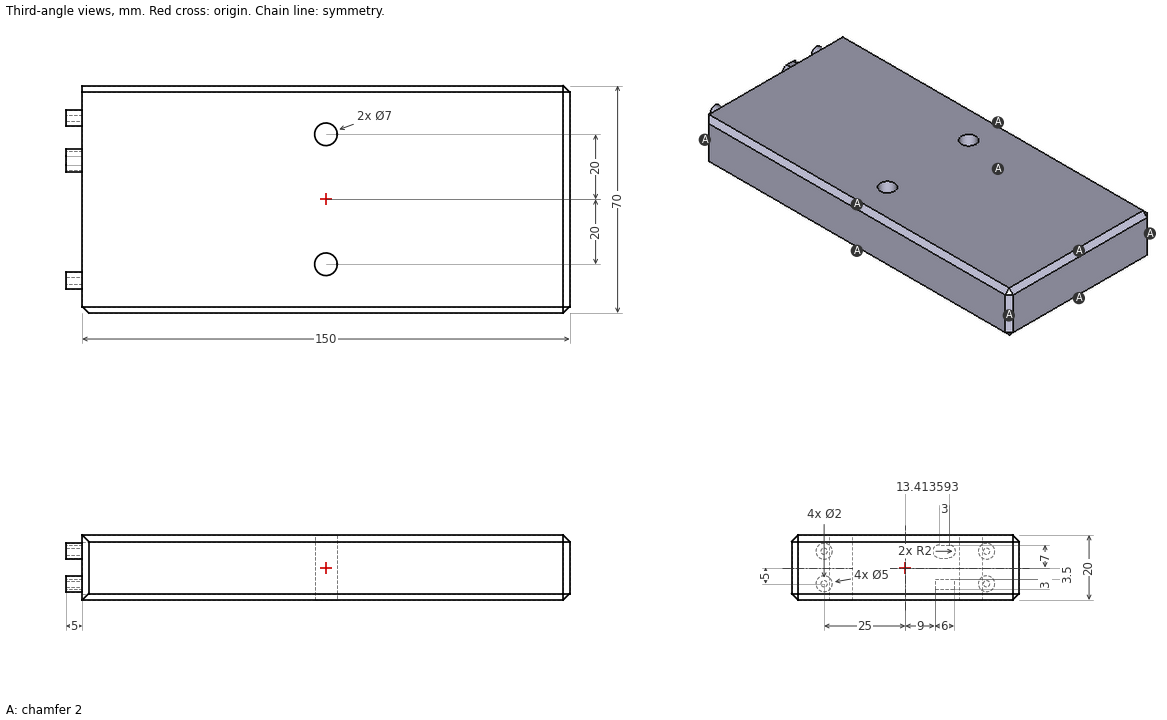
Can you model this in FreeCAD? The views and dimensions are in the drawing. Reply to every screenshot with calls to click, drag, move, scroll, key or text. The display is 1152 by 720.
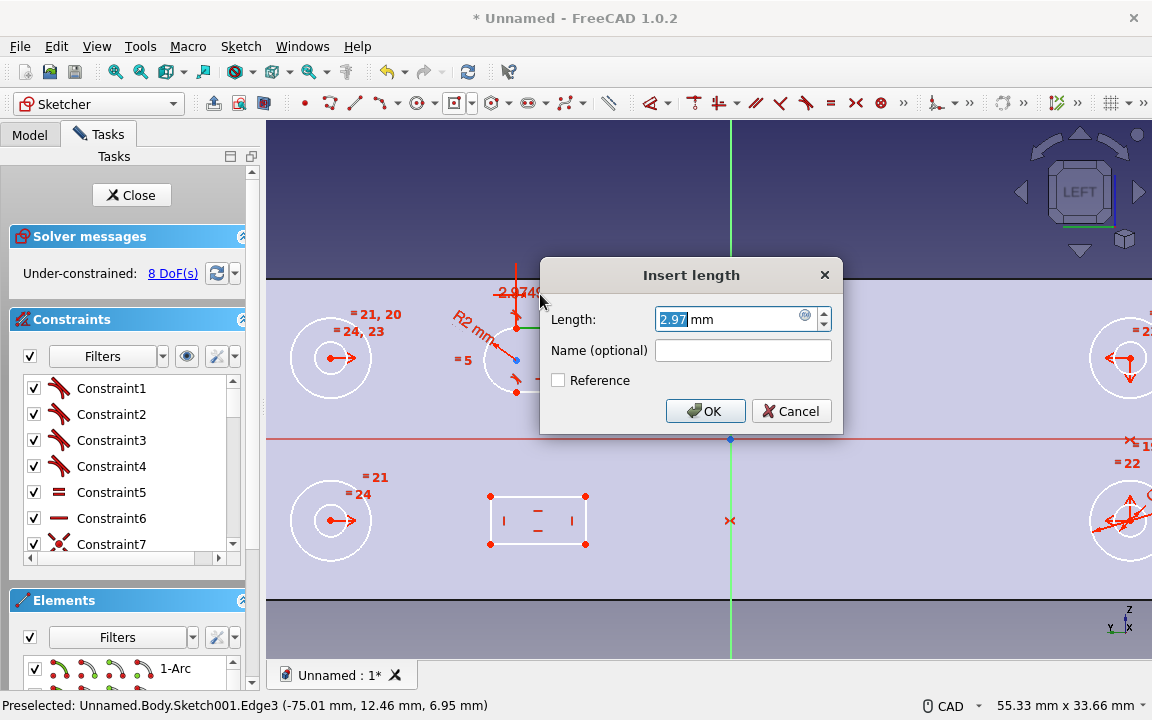
text(3)
key(Return)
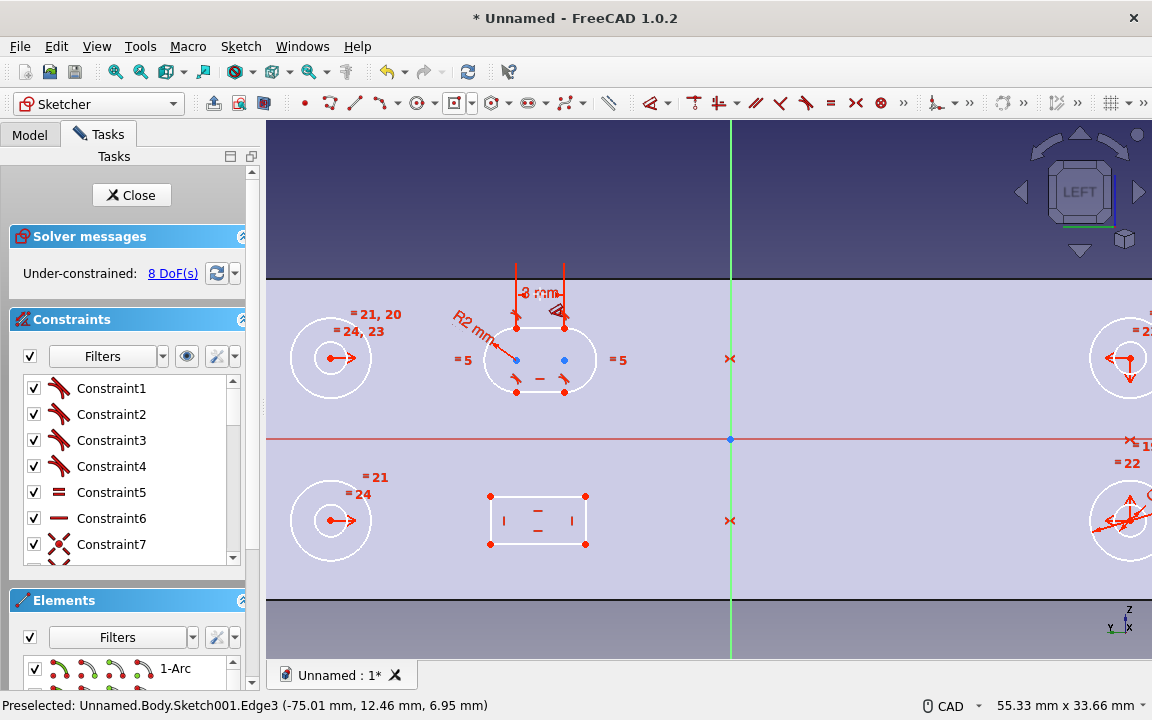
click(491, 511)
click(457, 520)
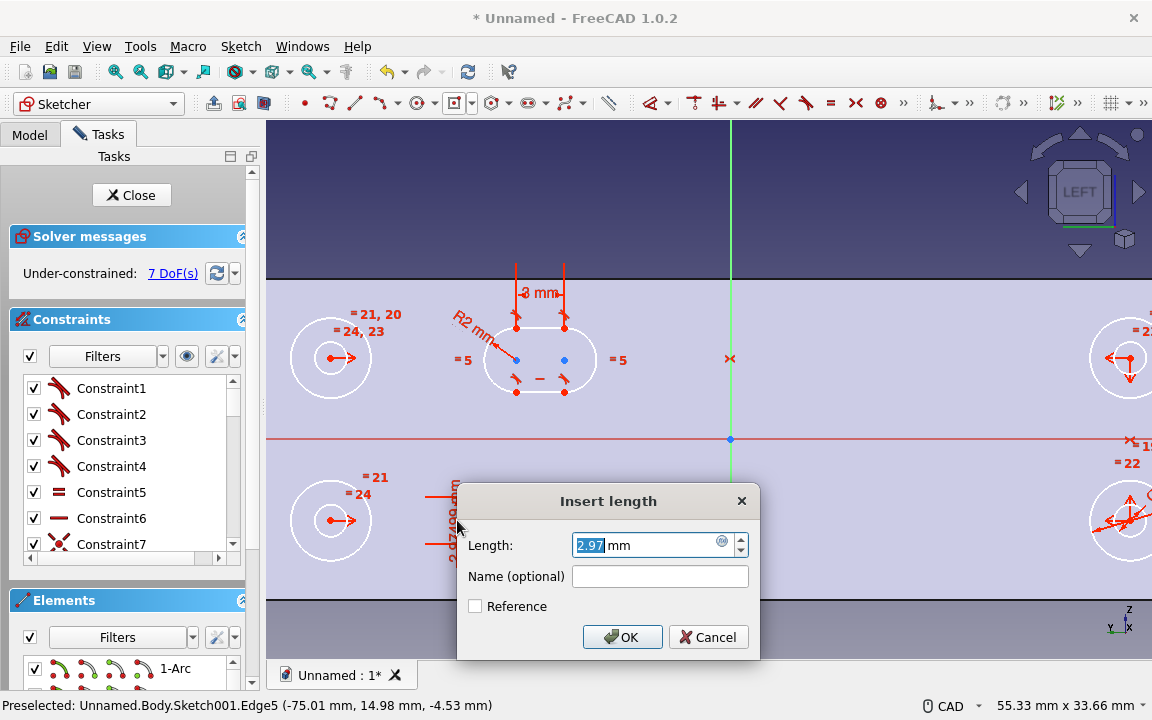
text(3)
key(Return)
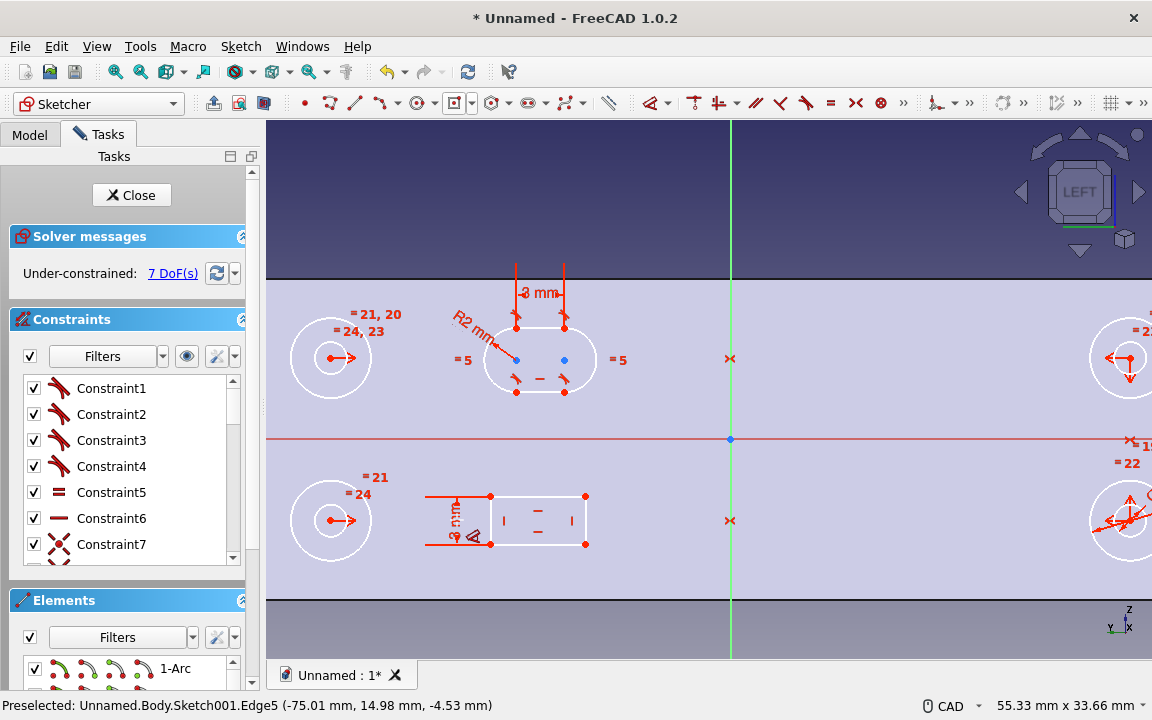
click(519, 545)
click(538, 579)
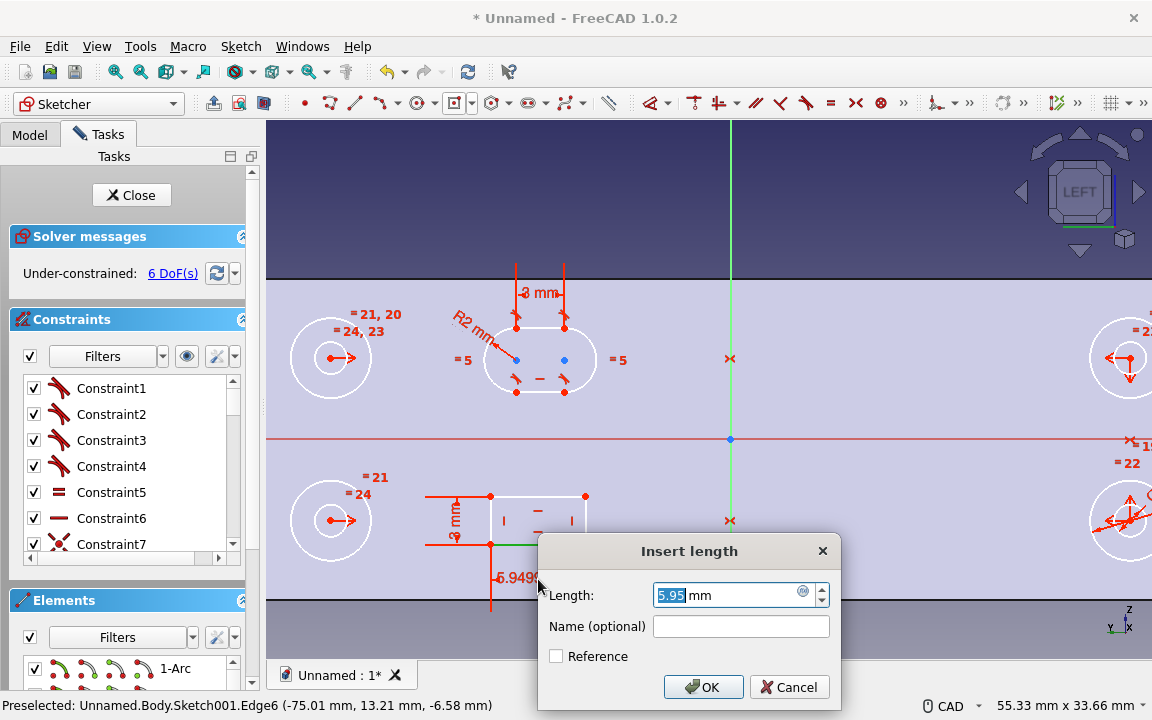
text(6)
key(Return)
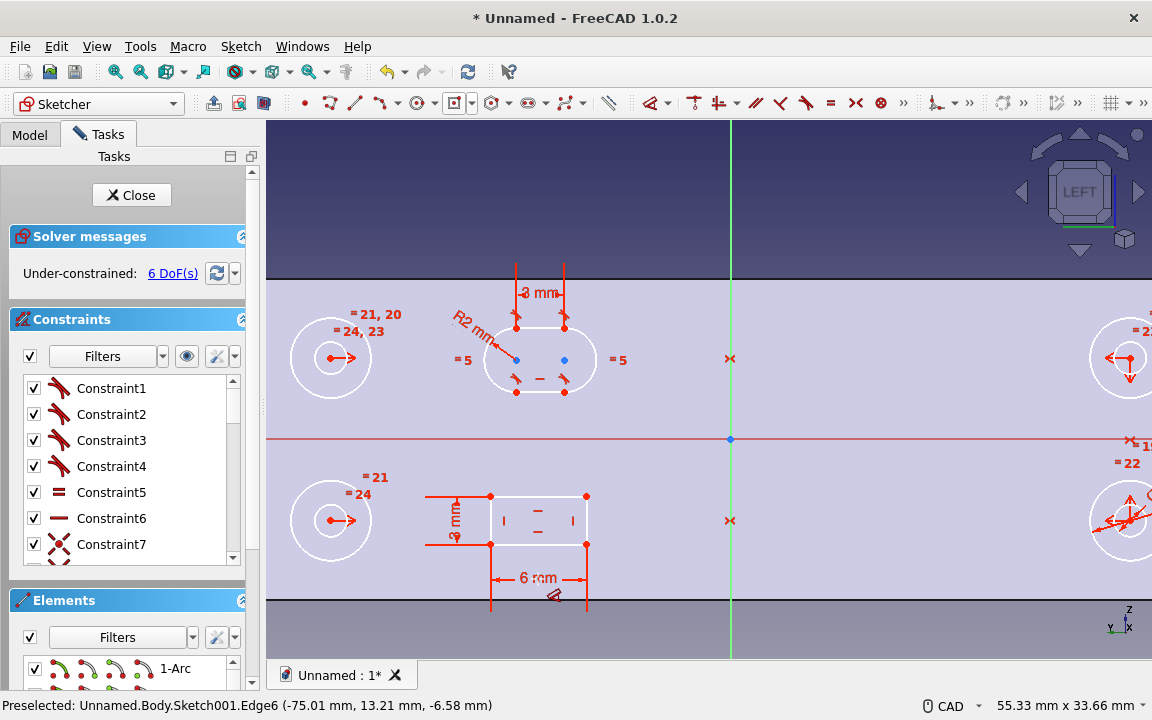
scroll(531, 329, down, 3)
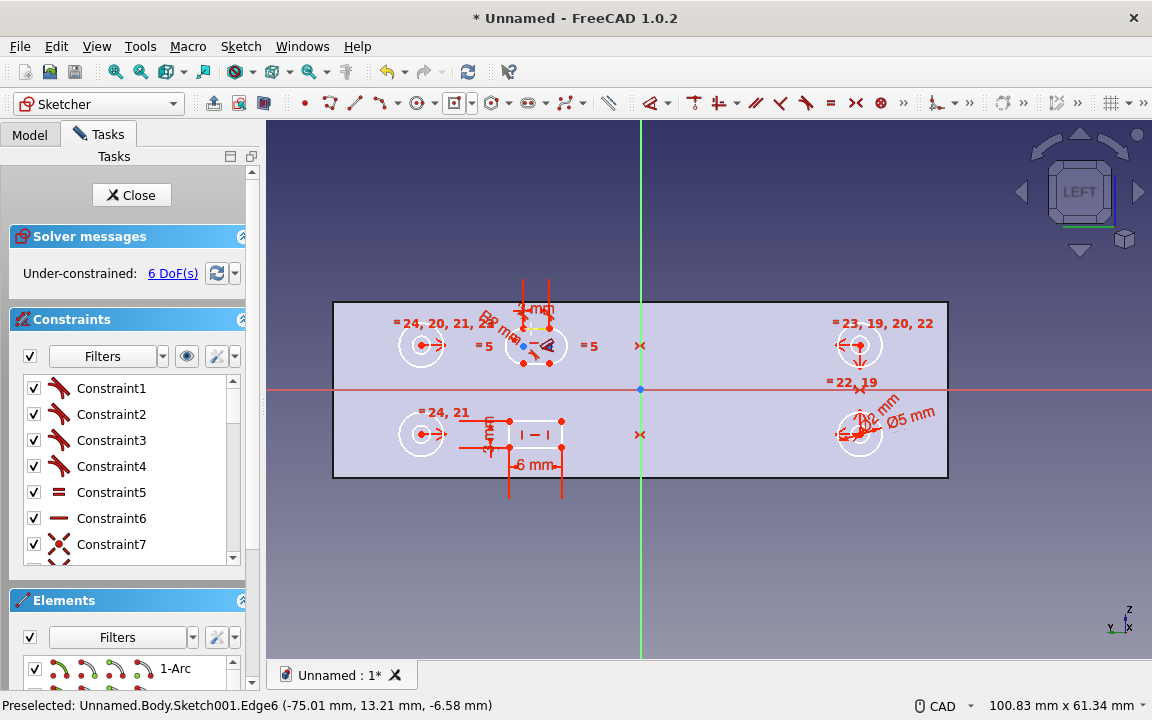
click(860, 434)
click(607, 412)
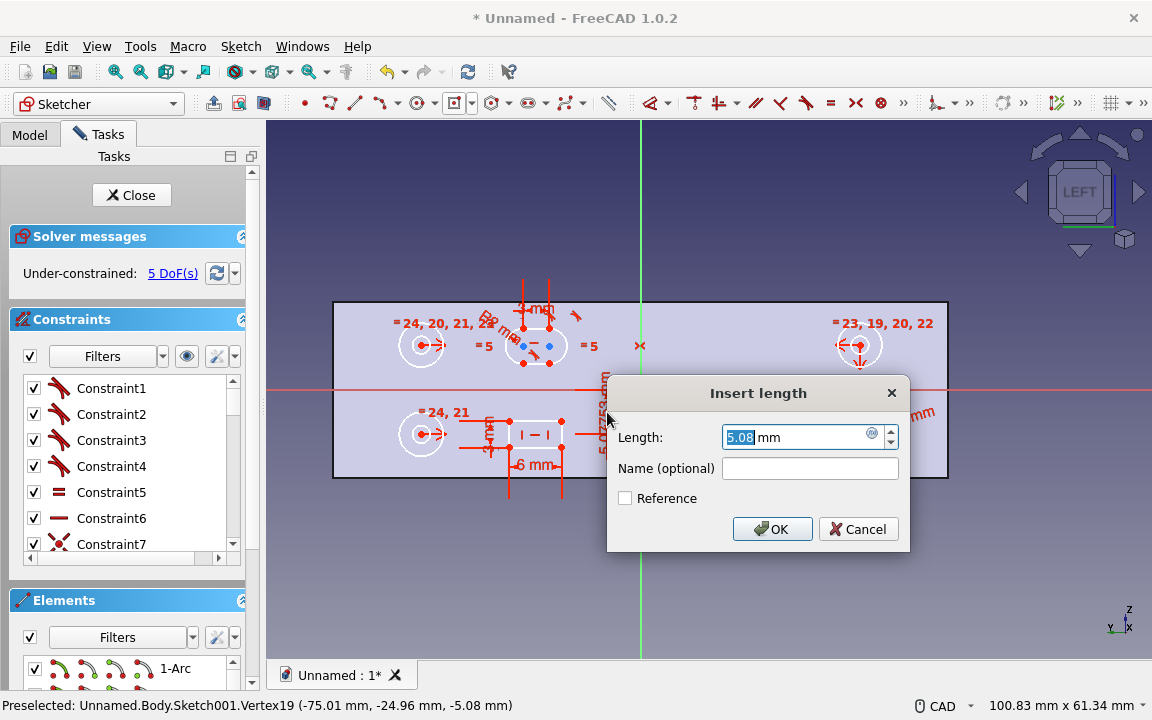
text(5)
key(Return)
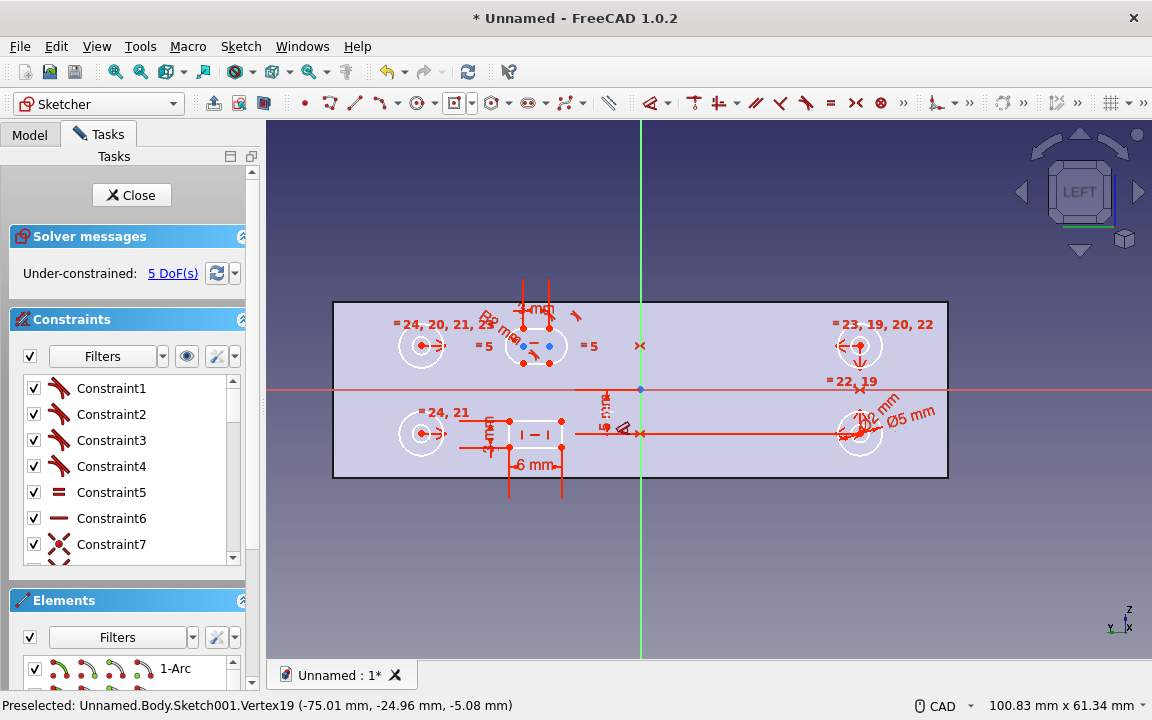
click(523, 329)
click(489, 359)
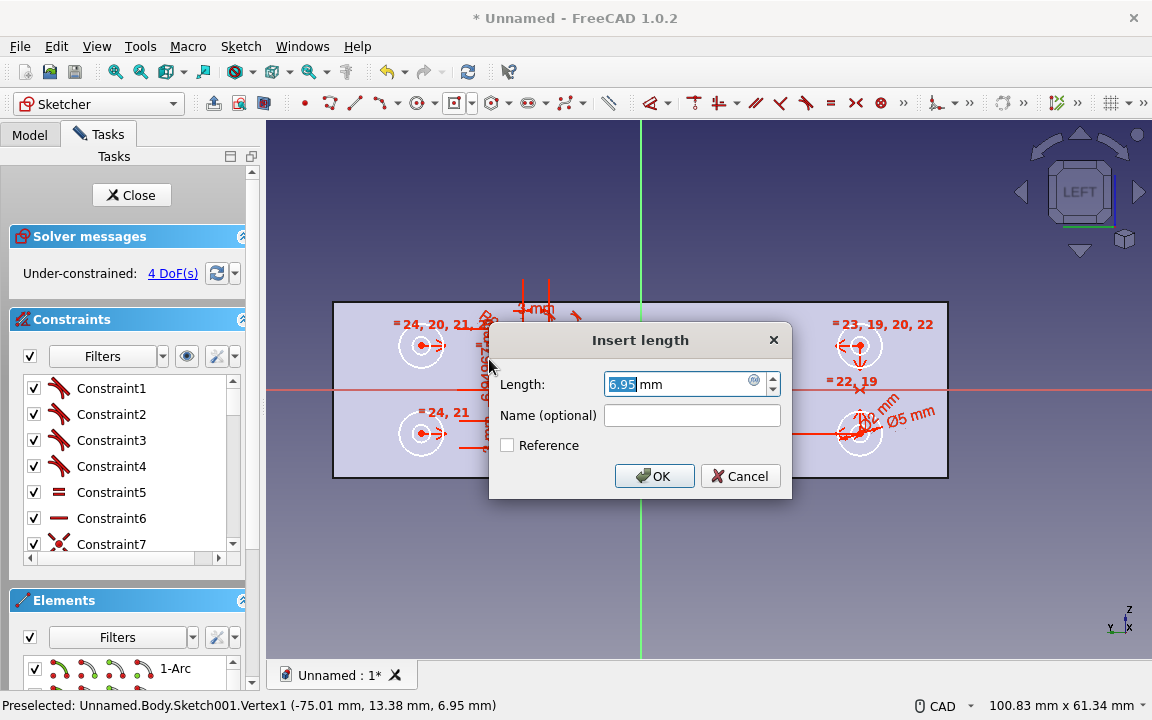
text(7)
key(Return)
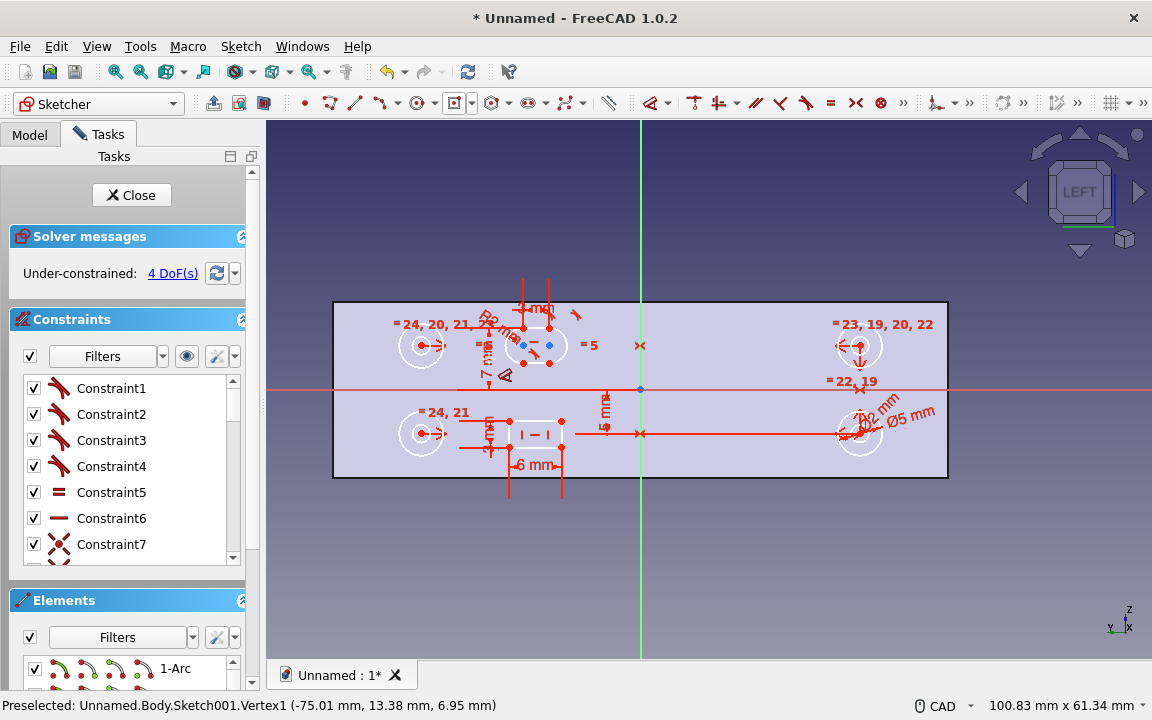
click(562, 448)
click(619, 482)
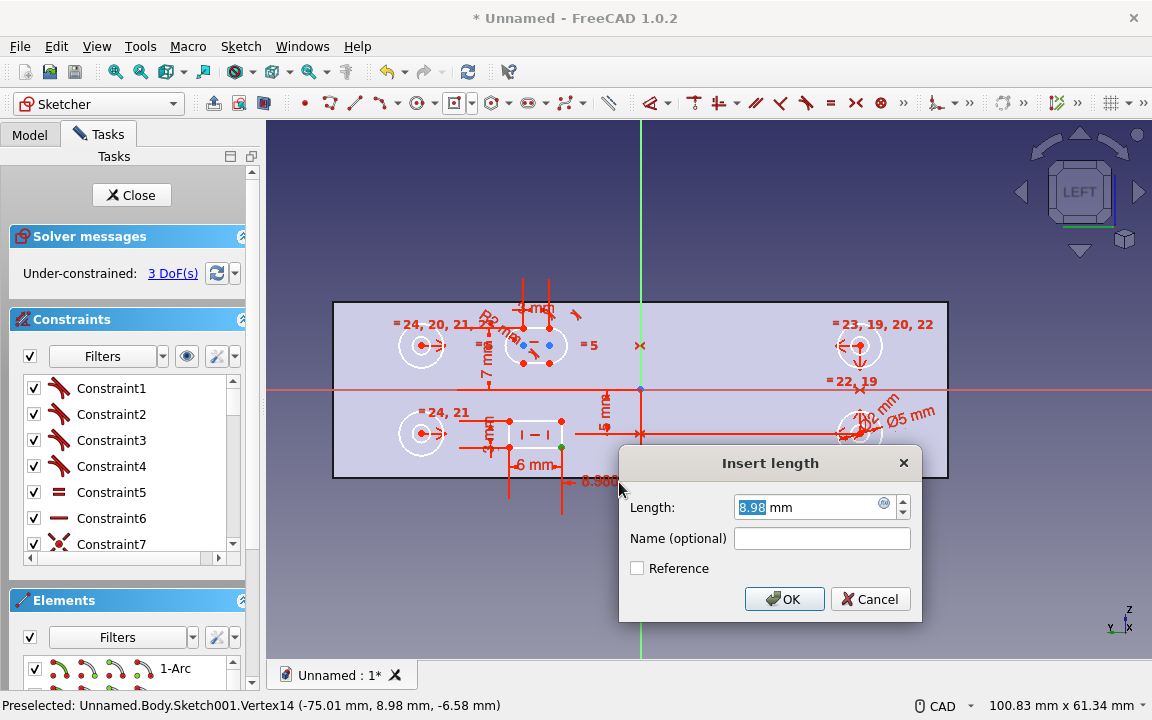
text(9)
key(Return)